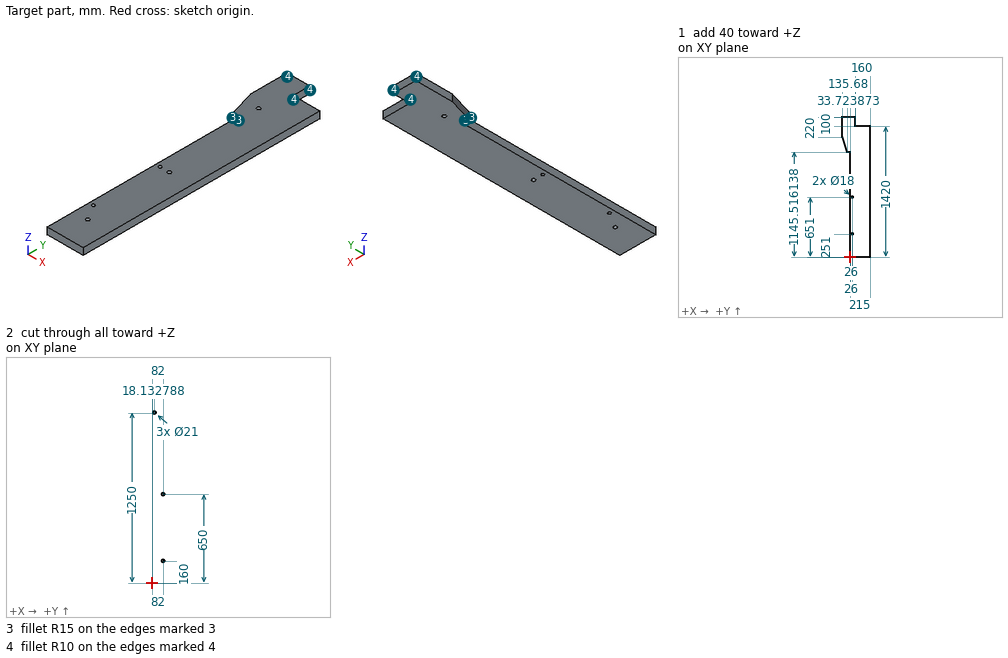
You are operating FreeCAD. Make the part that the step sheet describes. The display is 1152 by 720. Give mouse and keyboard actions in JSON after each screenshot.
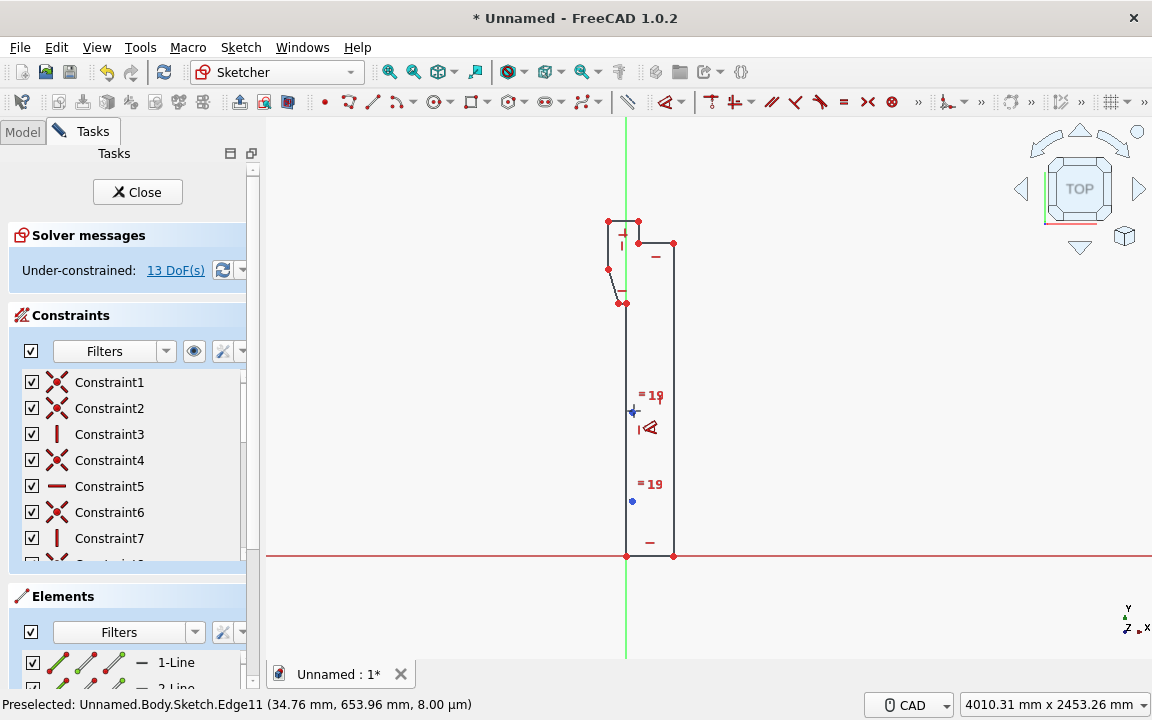
{"action": "scroll", "coordinate": [634, 499], "scroll_direction": "up", "scroll_amount": 12}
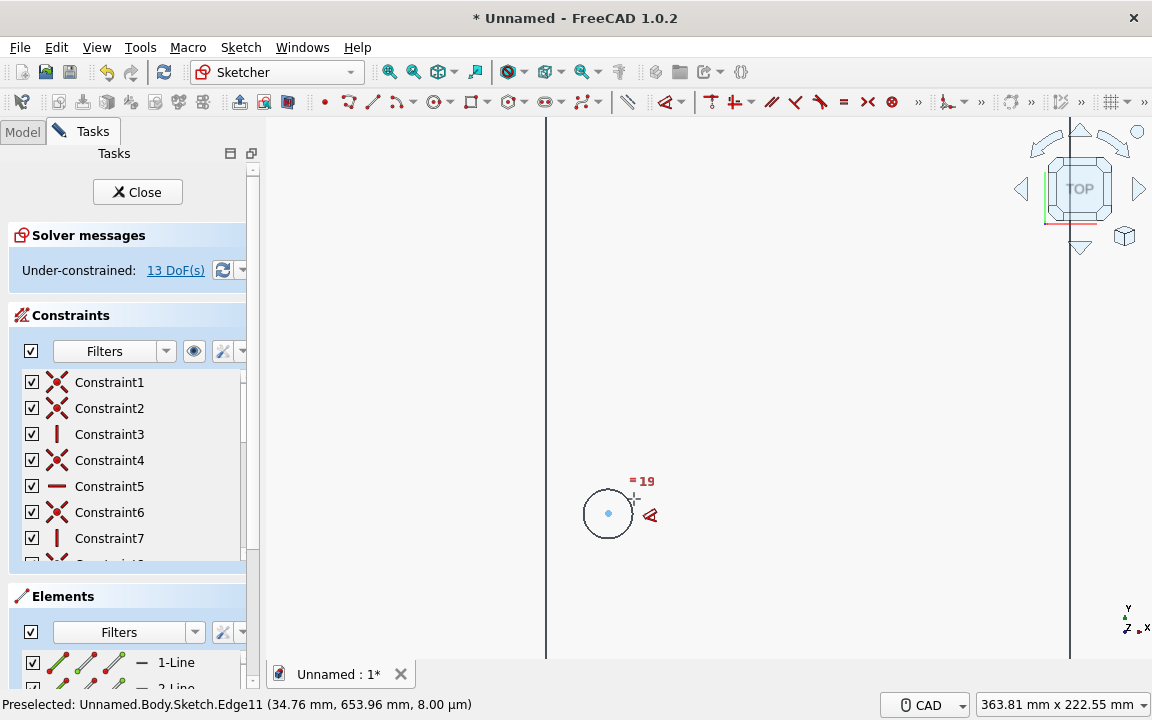
{"action": "left_click", "coordinate": [625, 497]}
{"action": "left_click", "coordinate": [648, 474]}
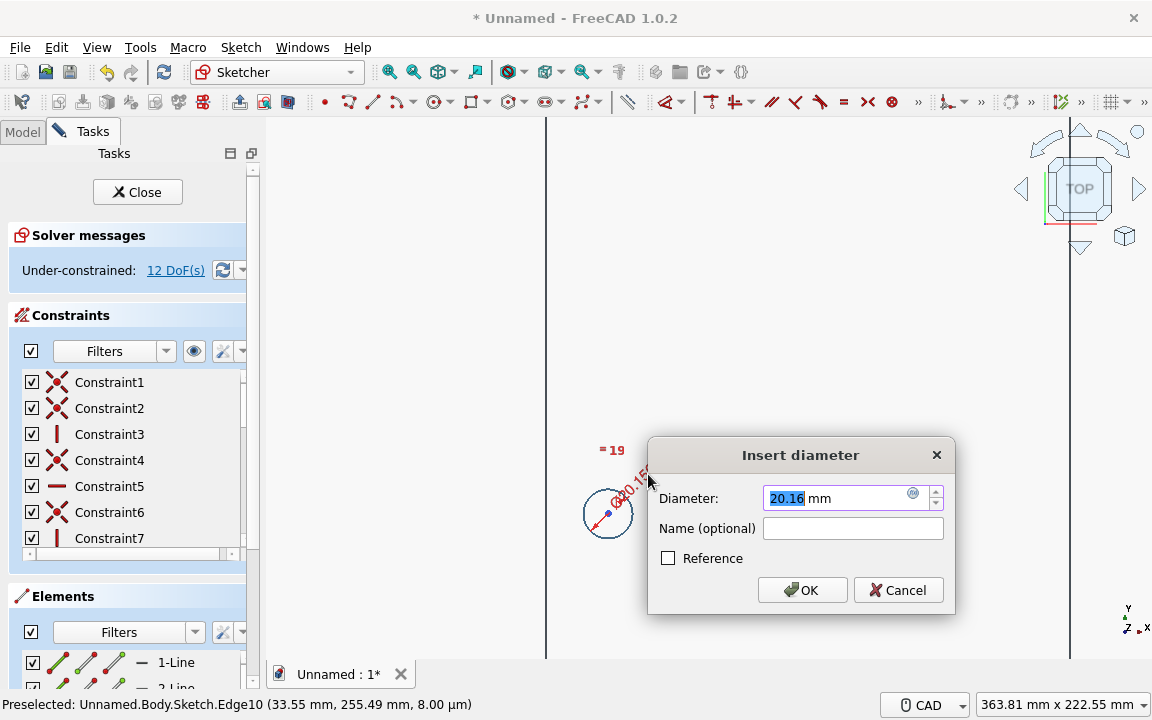
{"action": "type", "text": "18"}
{"action": "key", "text": "Return"}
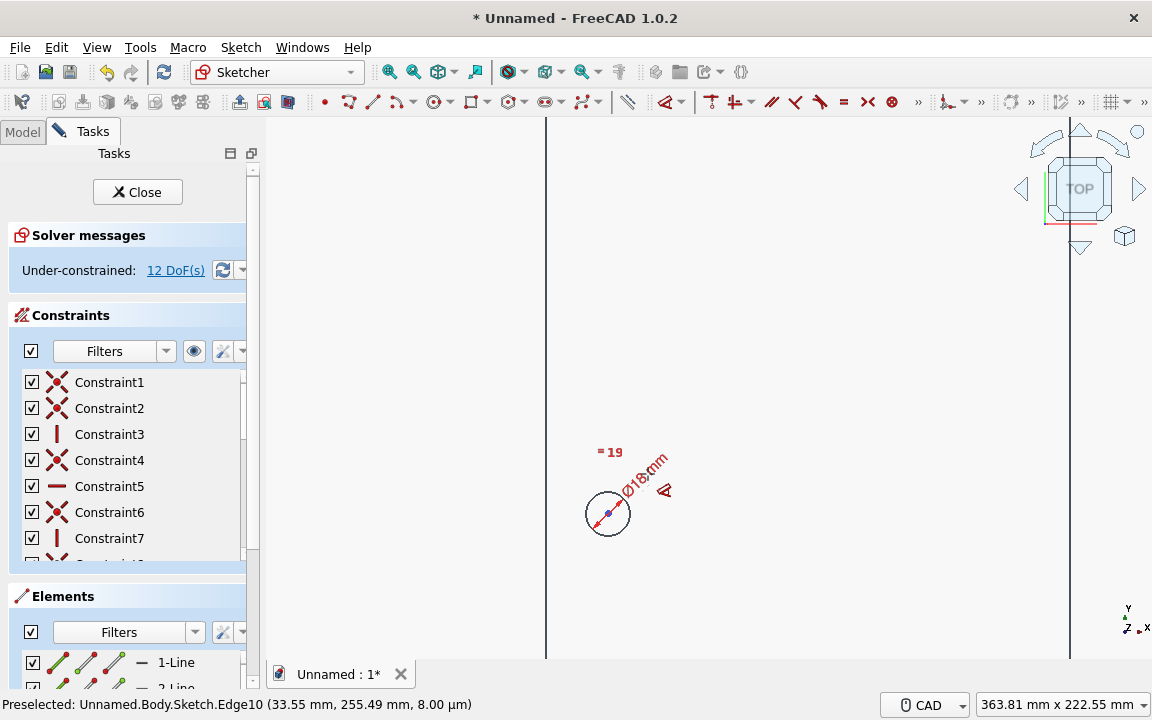
{"action": "left_click", "coordinate": [608, 514]}
{"action": "left_click", "coordinate": [577, 480]}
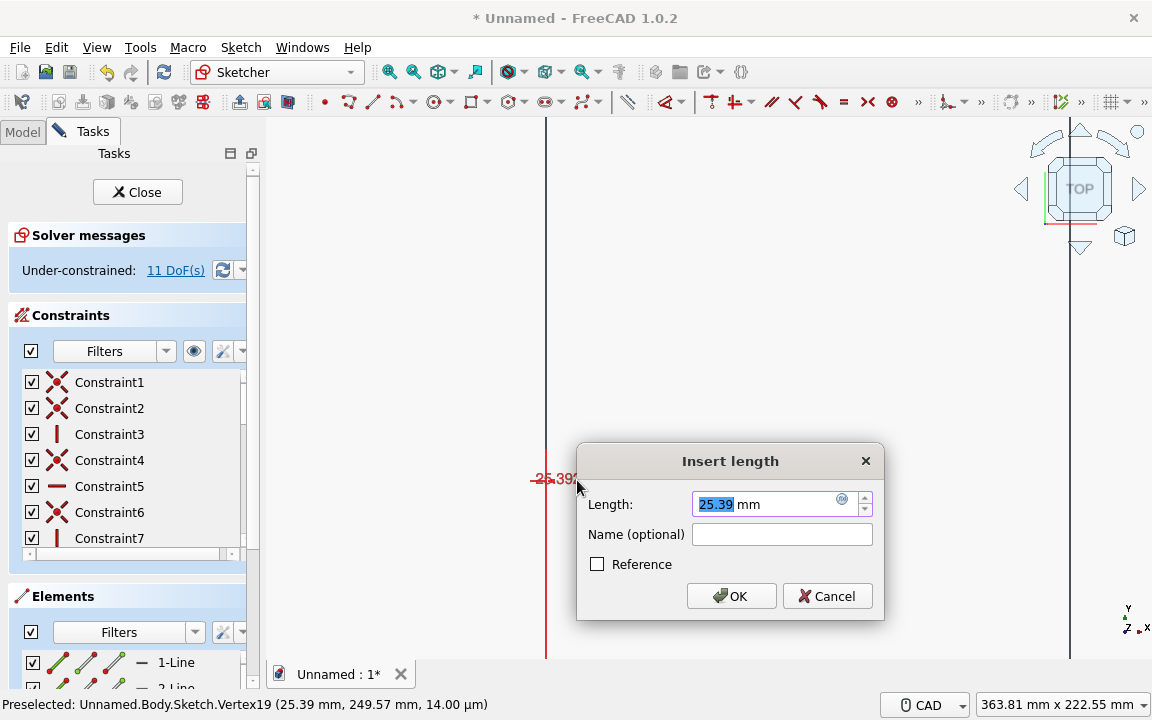
{"action": "type", "text": "26"}
{"action": "key", "text": "Return"}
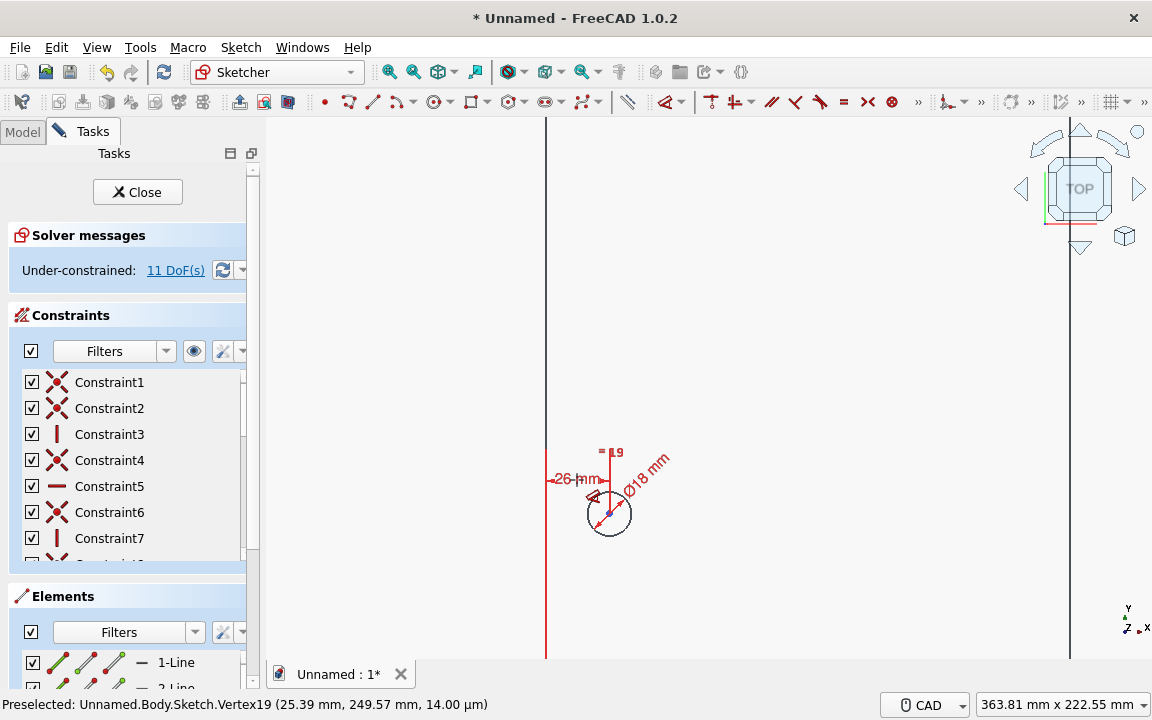
{"action": "scroll", "coordinate": [634, 499], "scroll_direction": "down", "scroll_amount": 12}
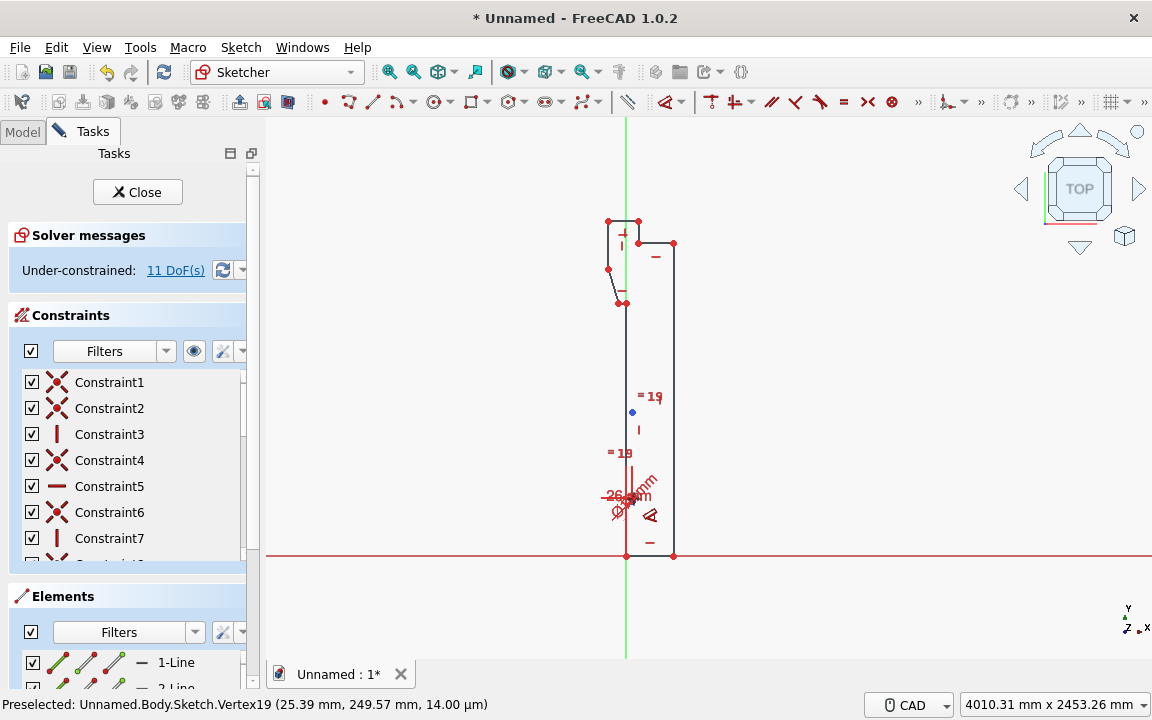
{"action": "scroll", "coordinate": [632, 413], "scroll_direction": "up", "scroll_amount": 10}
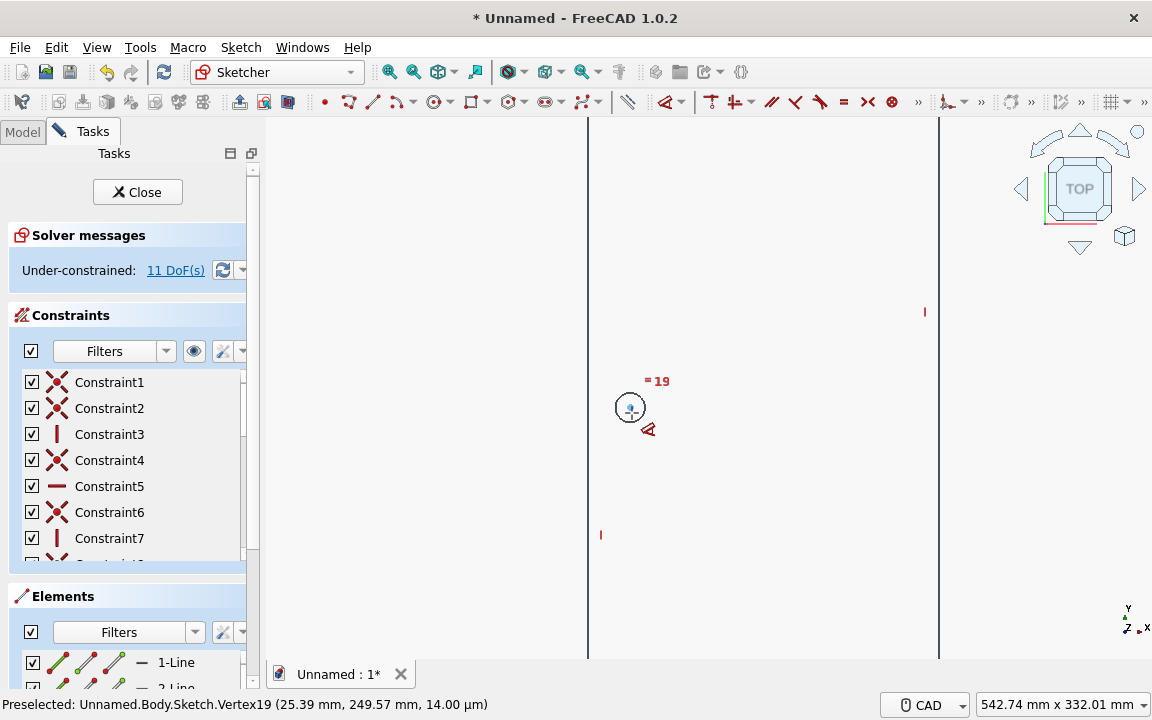
{"action": "left_click", "coordinate": [630, 408]}
{"action": "left_click", "coordinate": [609, 374]}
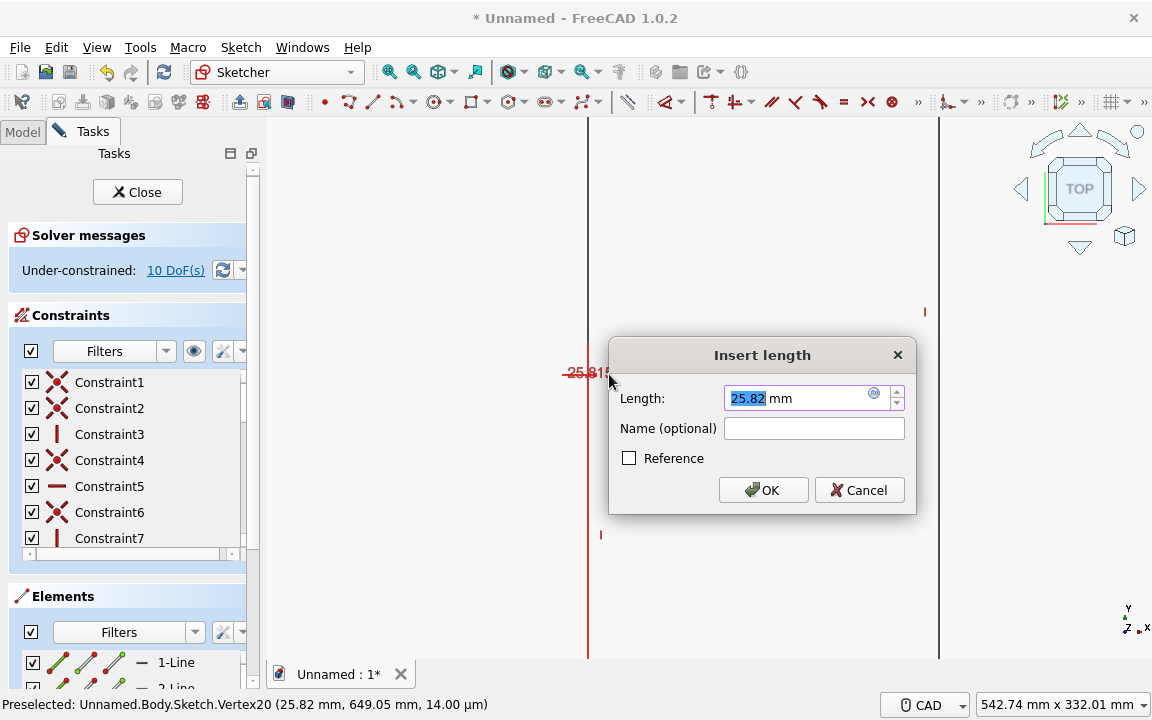
{"action": "type", "text": "26"}
{"action": "key", "text": "Return"}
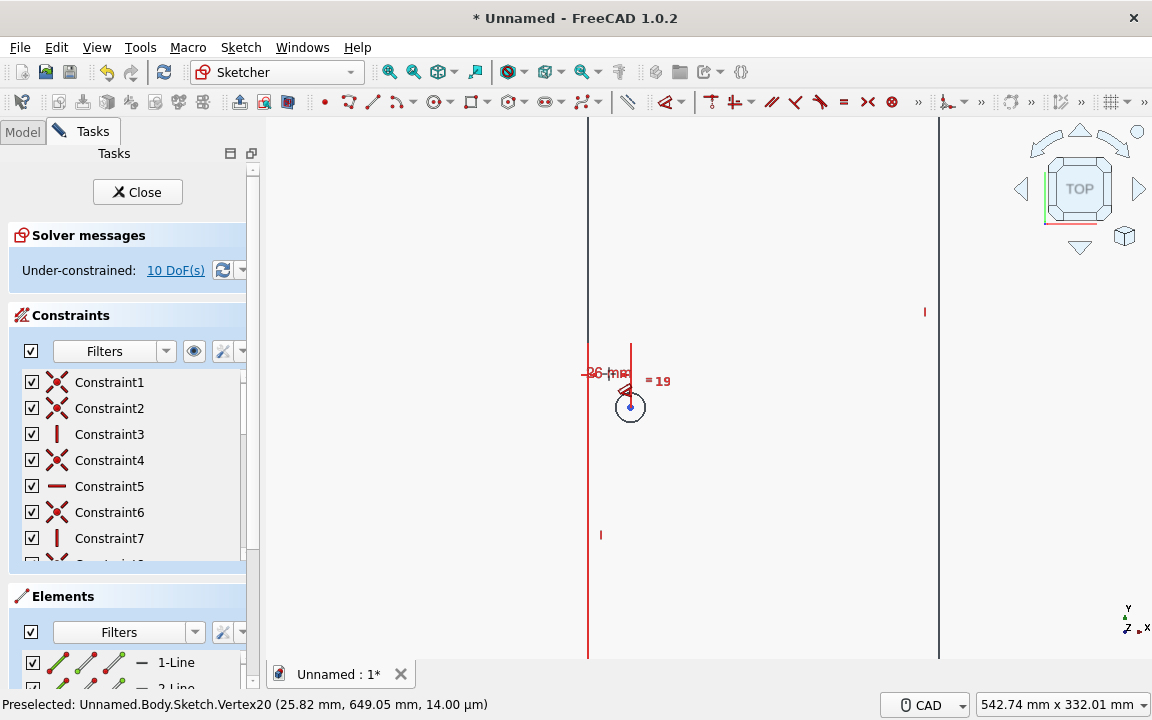
{"action": "scroll", "coordinate": [632, 413], "scroll_direction": "down", "scroll_amount": 10}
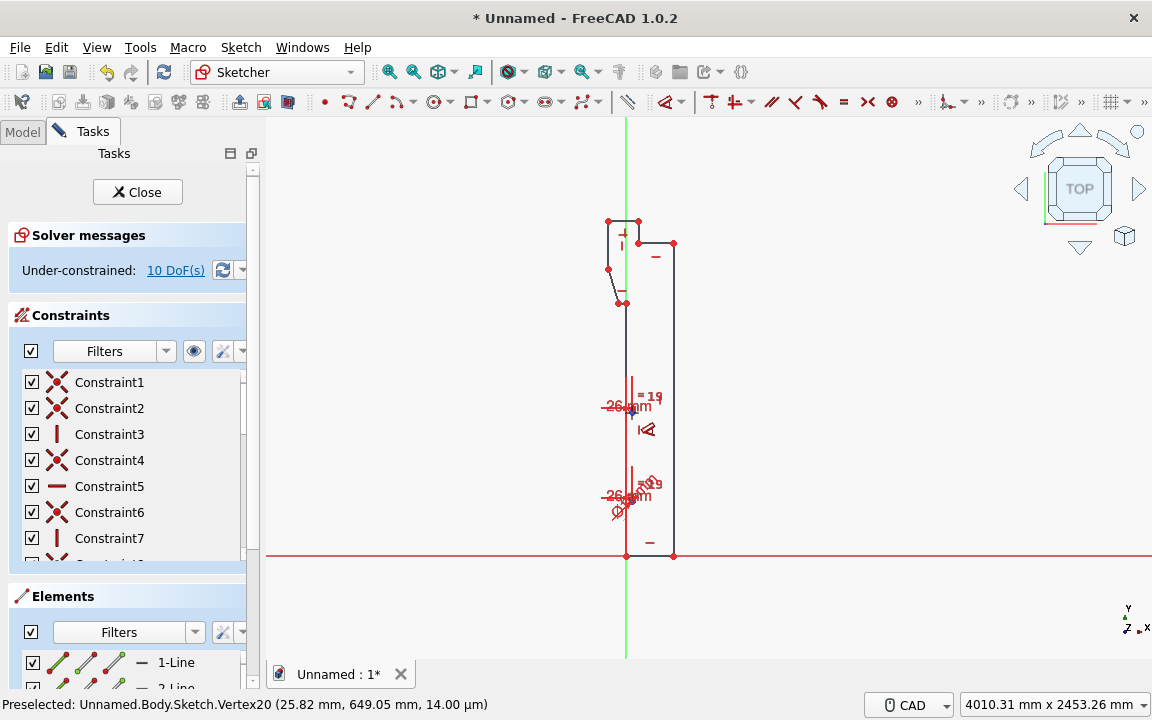
{"action": "left_click", "coordinate": [641, 556]}
{"action": "left_click", "coordinate": [650, 590]}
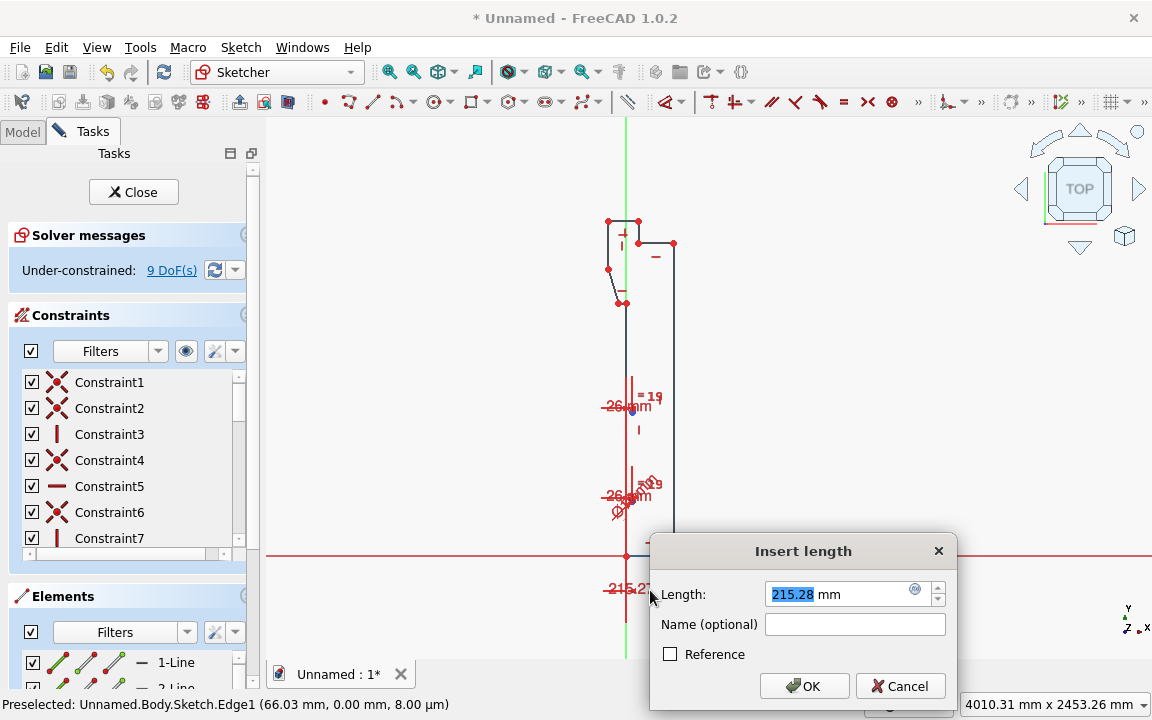
{"action": "type", "text": "215"}
{"action": "key", "text": "Return"}